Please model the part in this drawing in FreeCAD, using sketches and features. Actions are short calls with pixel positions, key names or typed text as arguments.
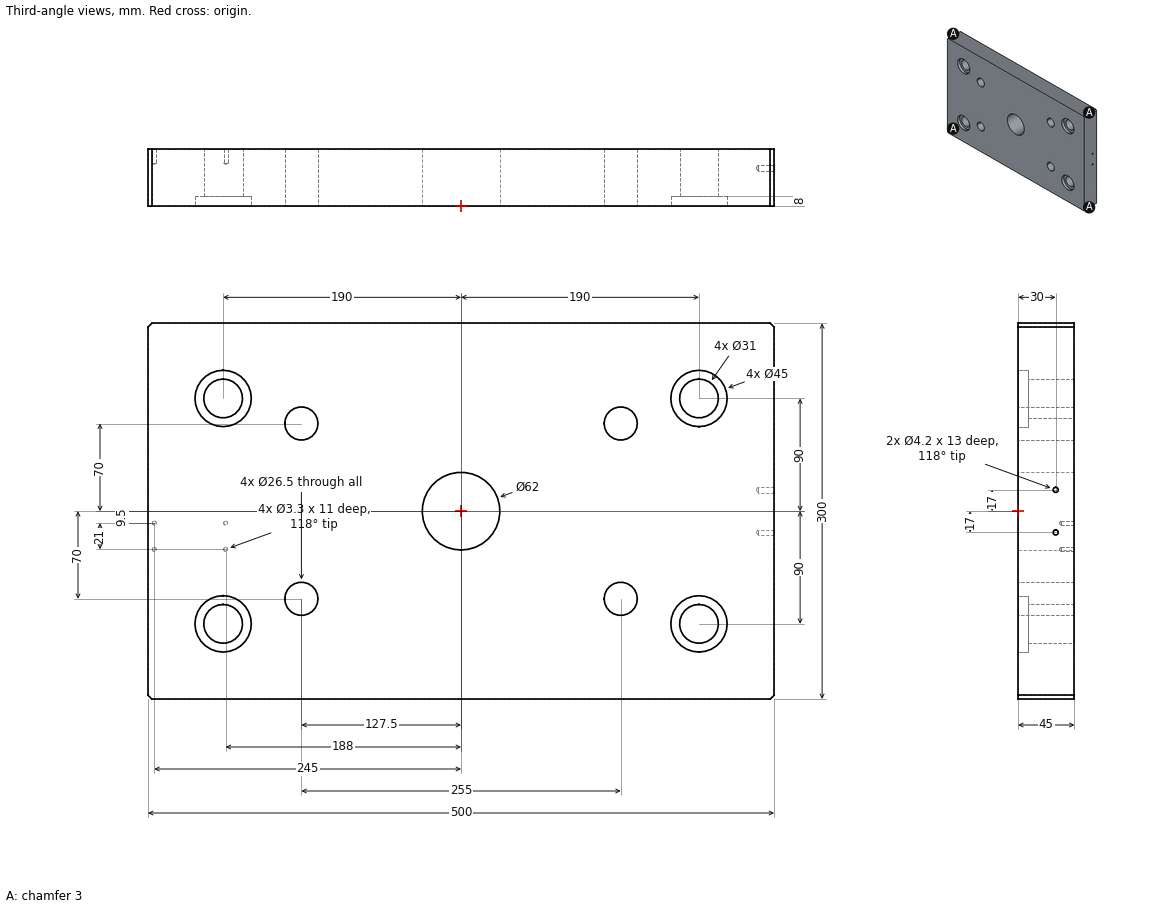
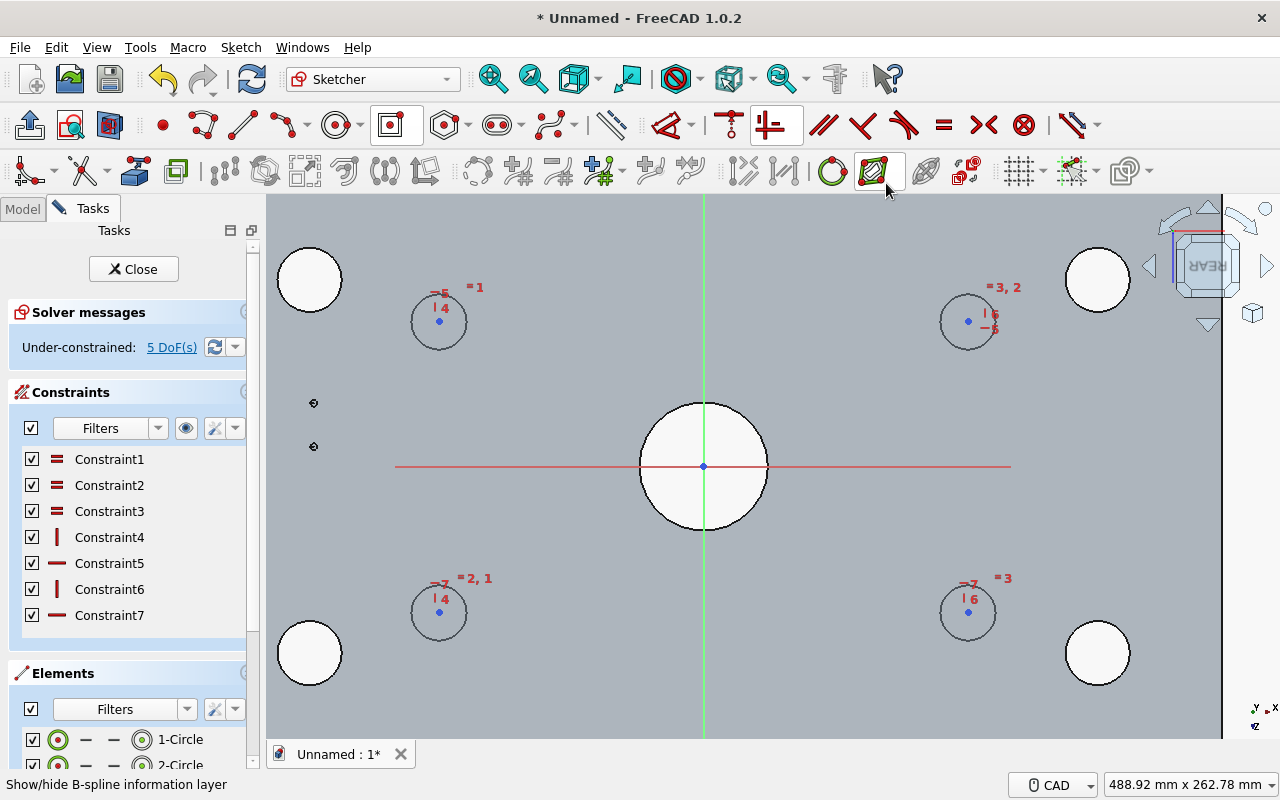
click(666, 126)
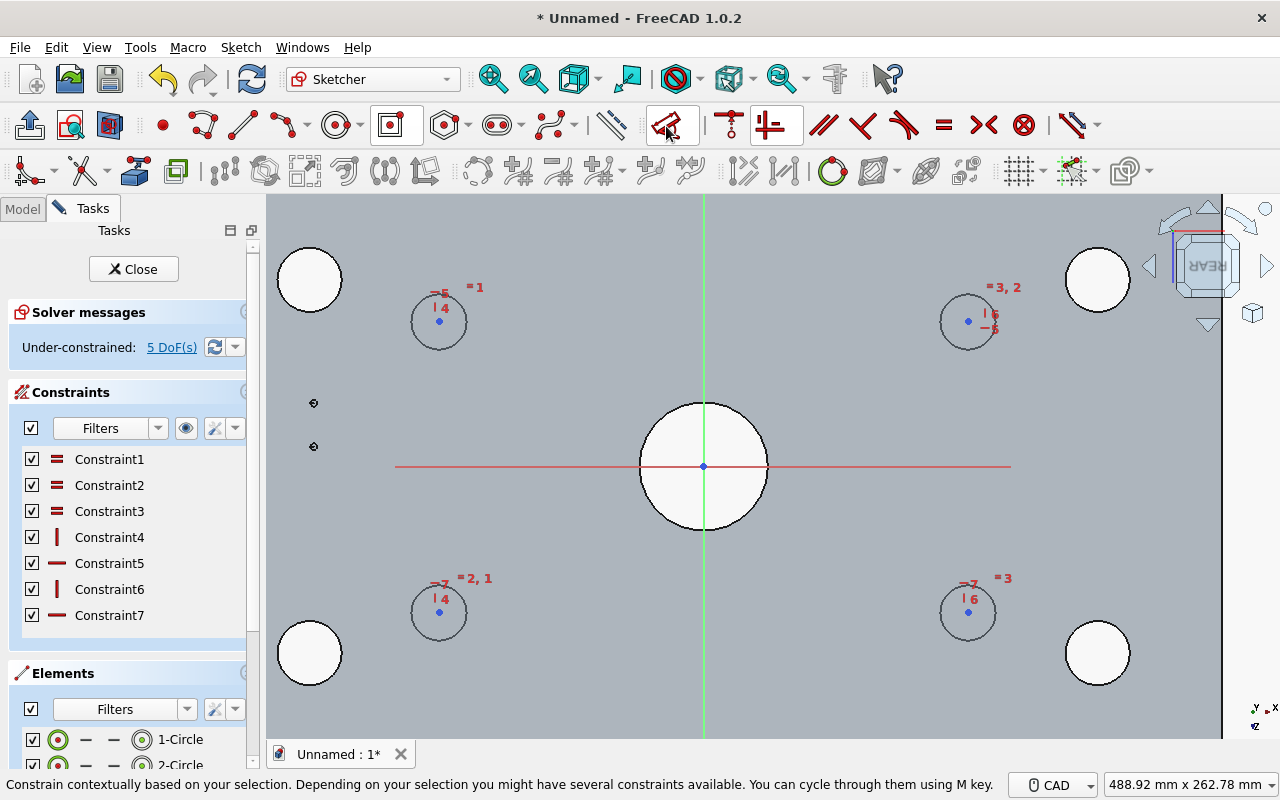
click(458, 302)
click(480, 279)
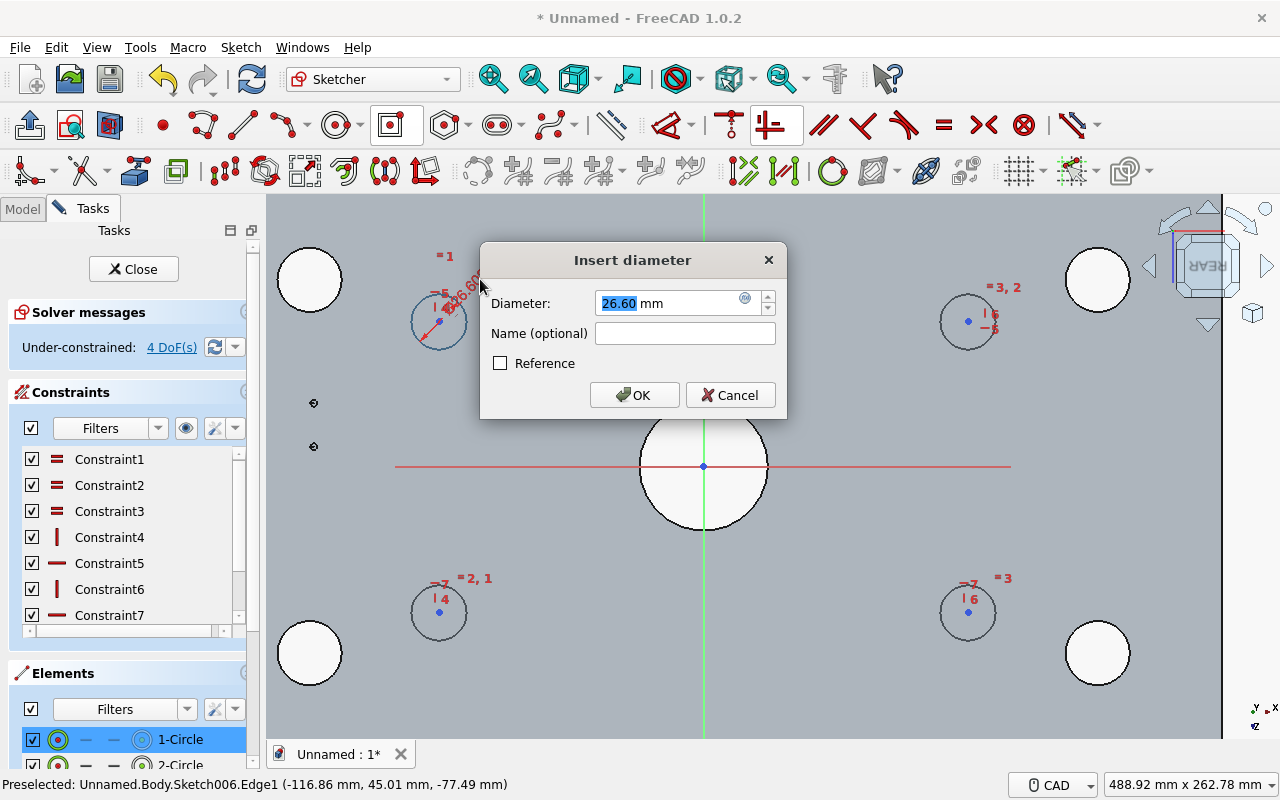
text(26.5)
key(Return)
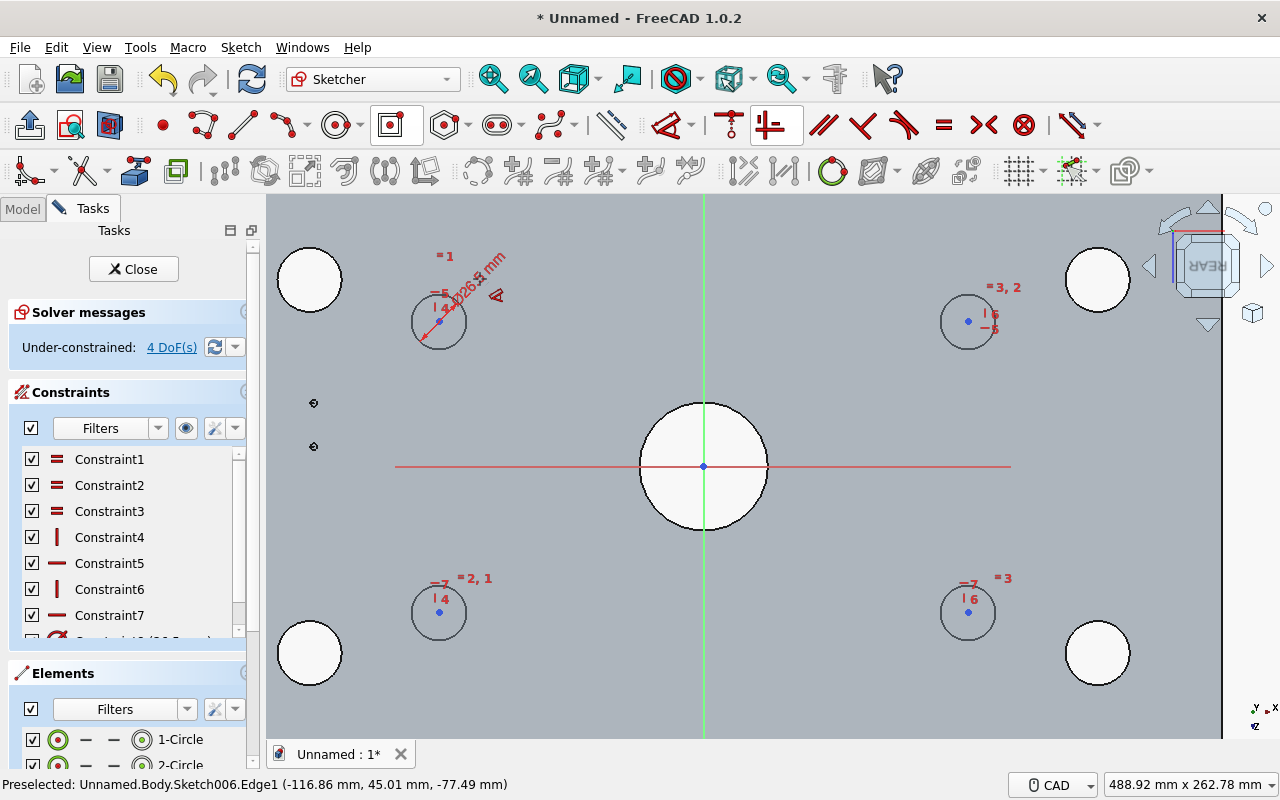
click(439, 322)
click(405, 394)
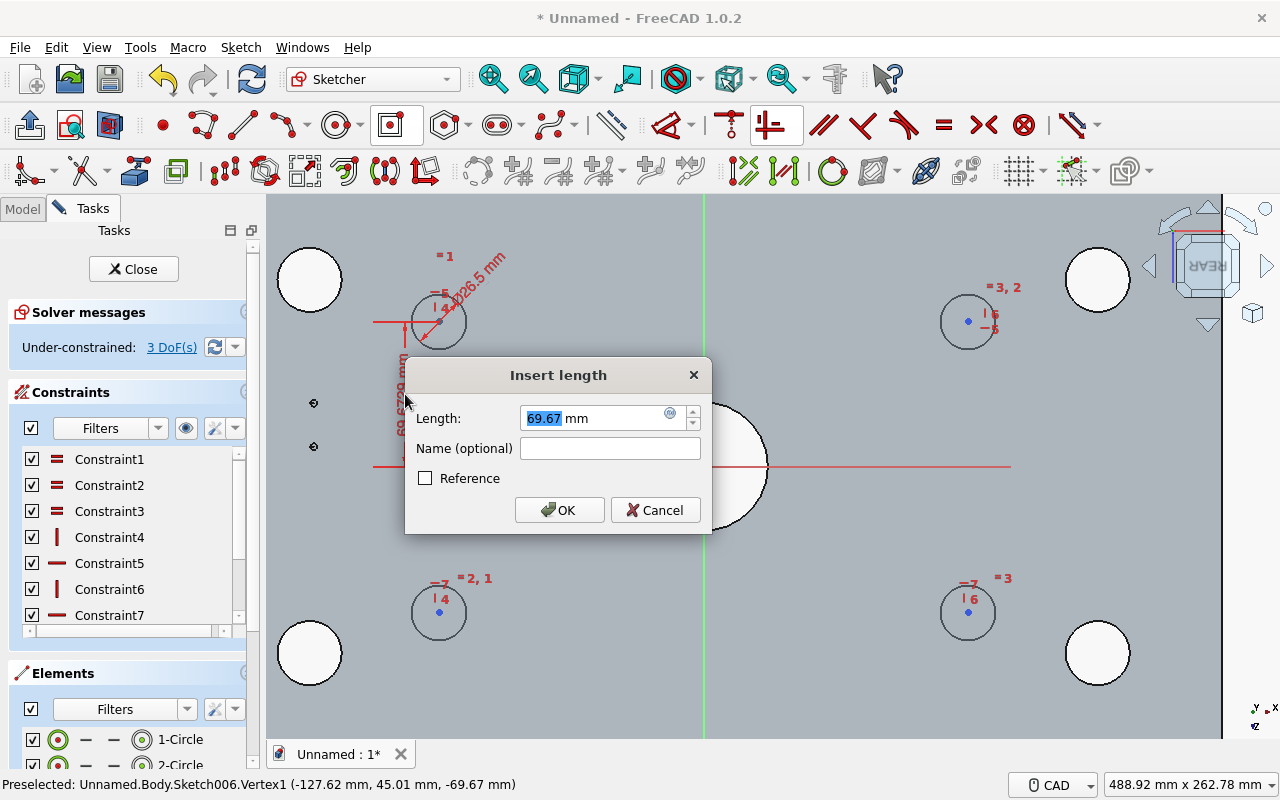
text(70)
key(Return)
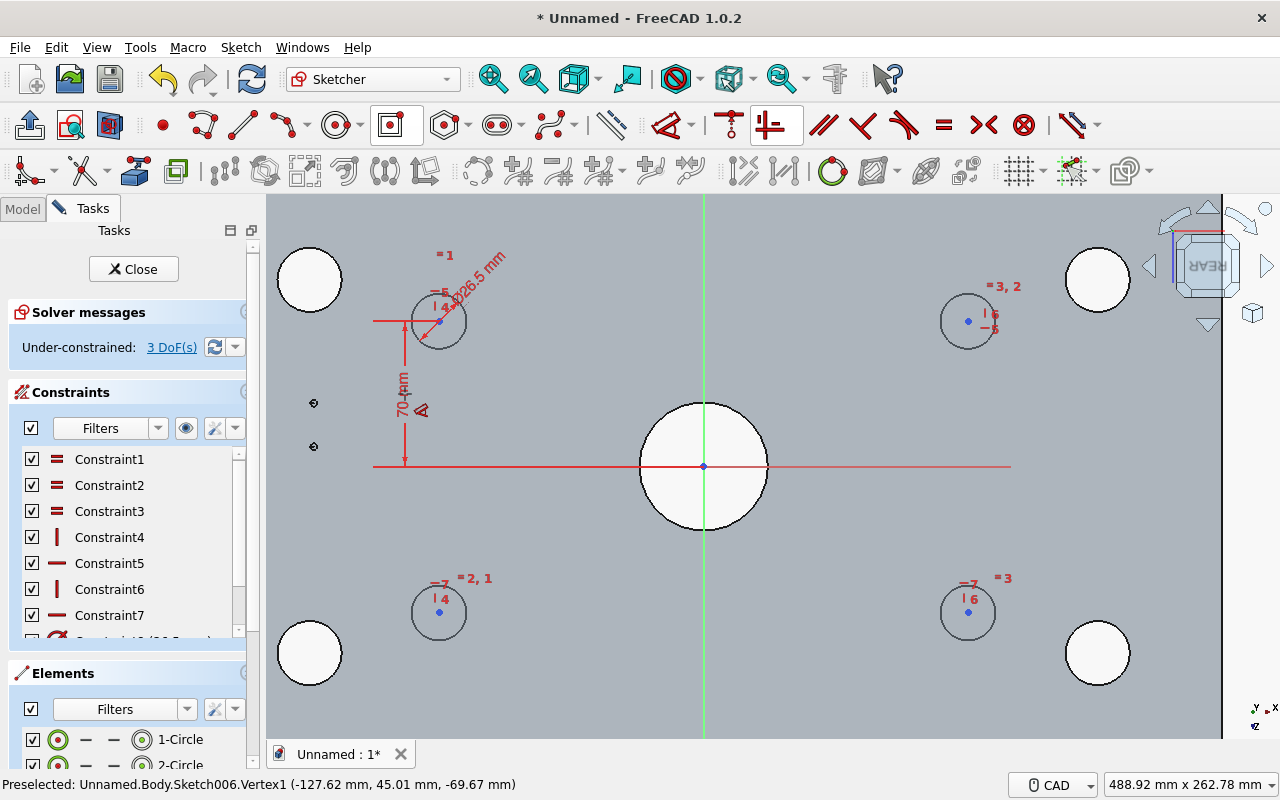
click(439, 613)
click(405, 540)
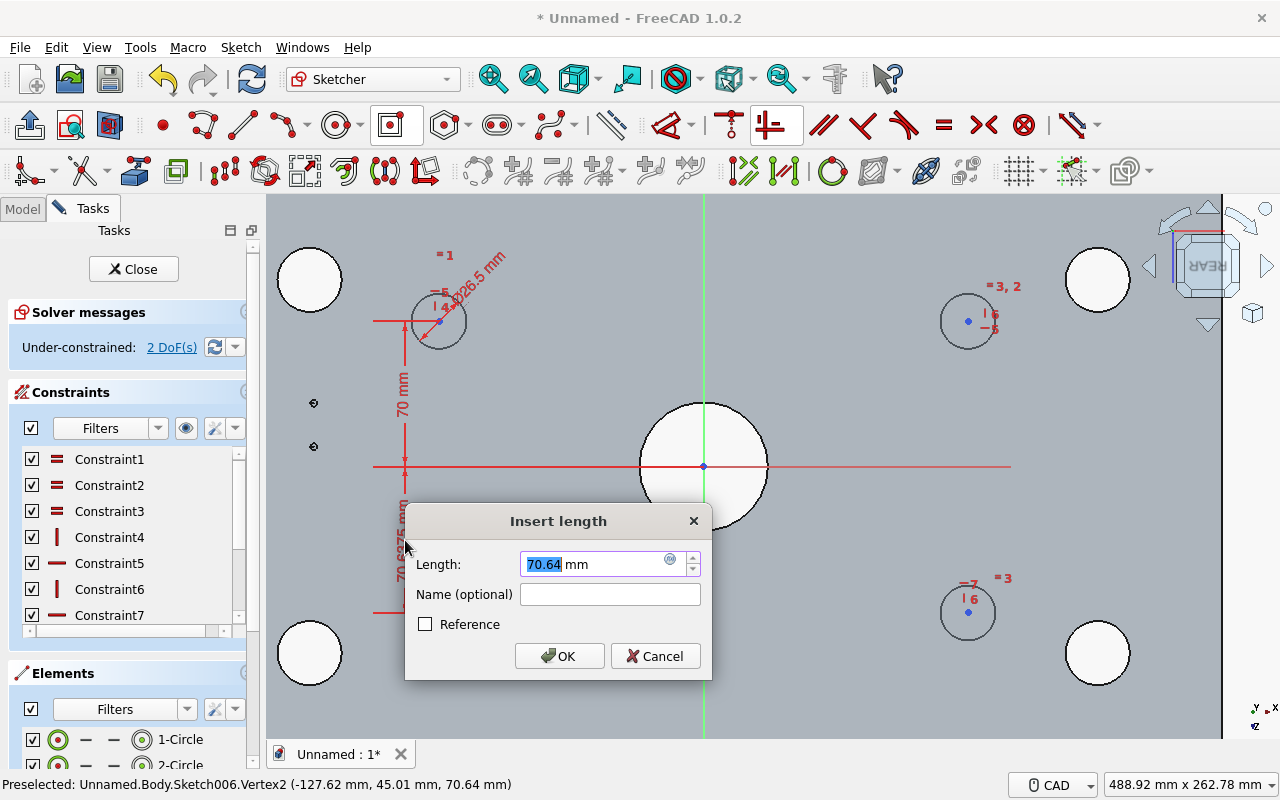
text(70)
key(Return)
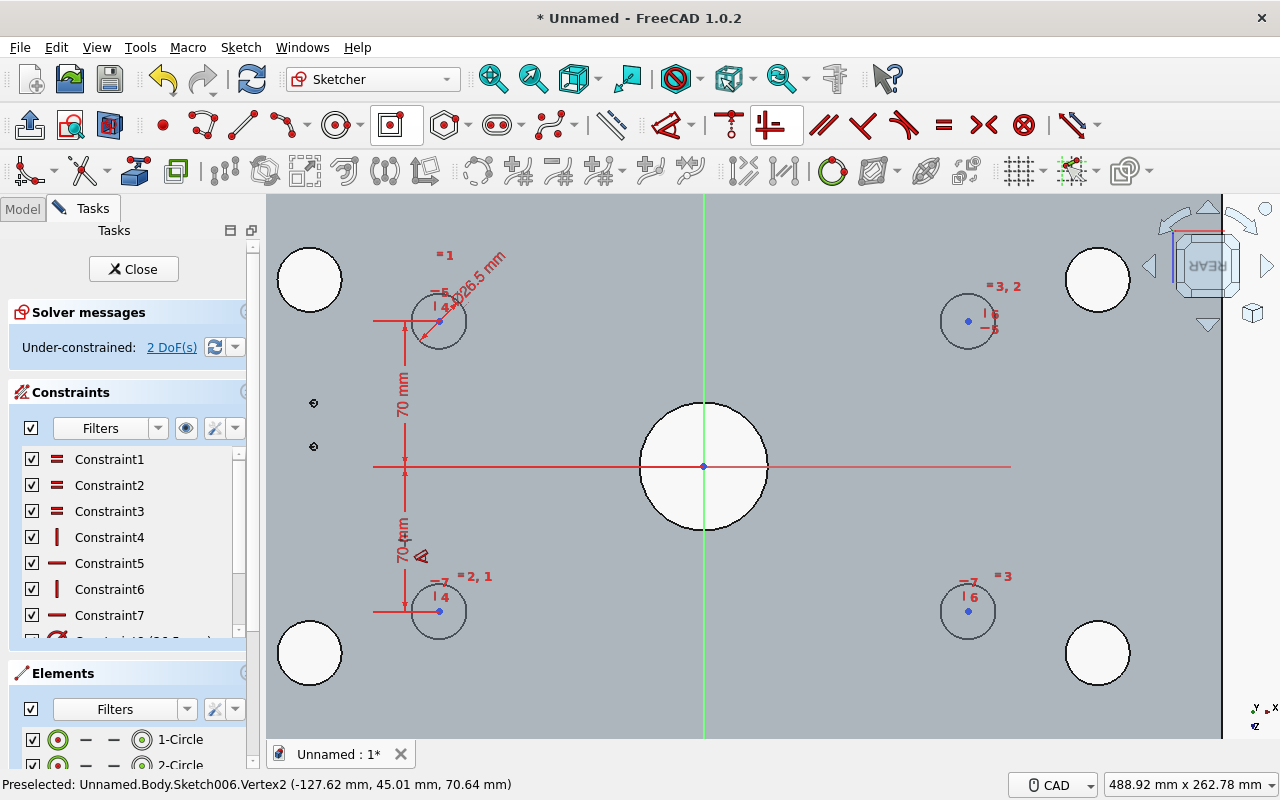
click(439, 321)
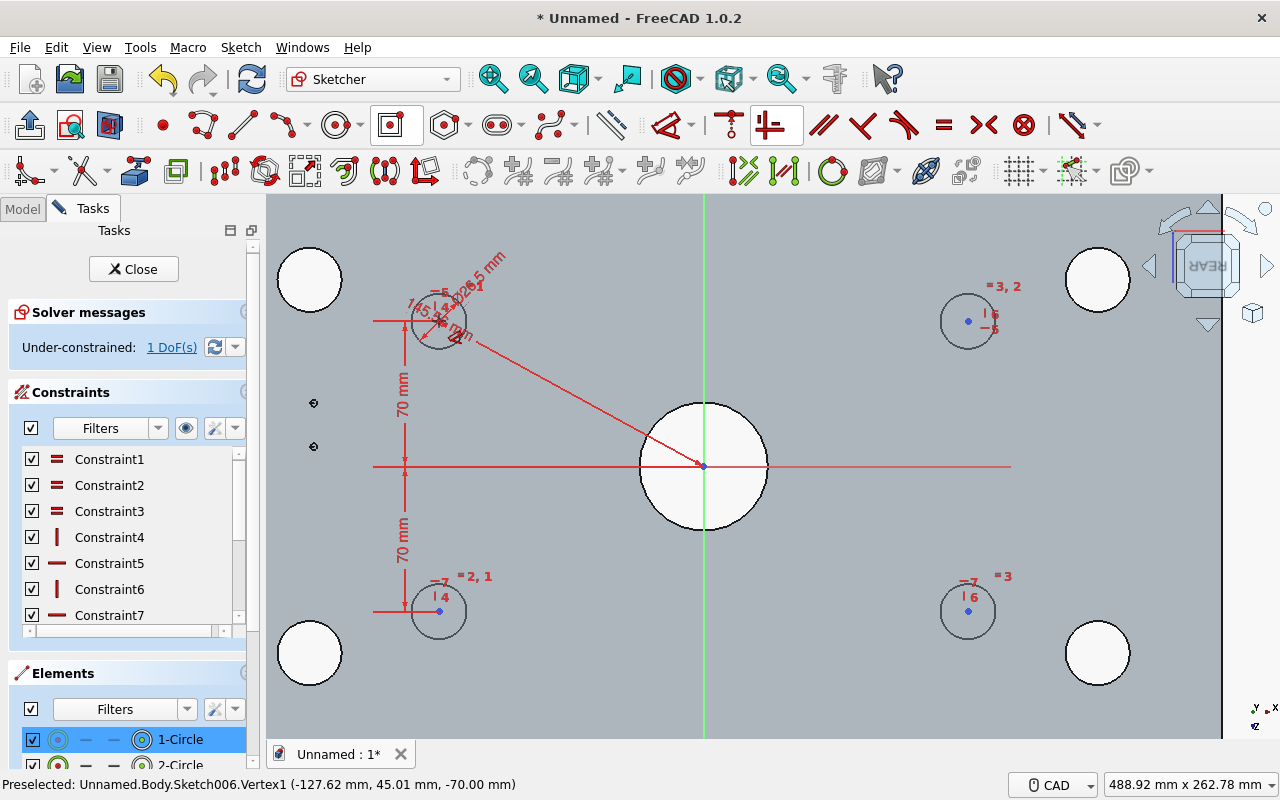
click(968, 321)
click(582, 287)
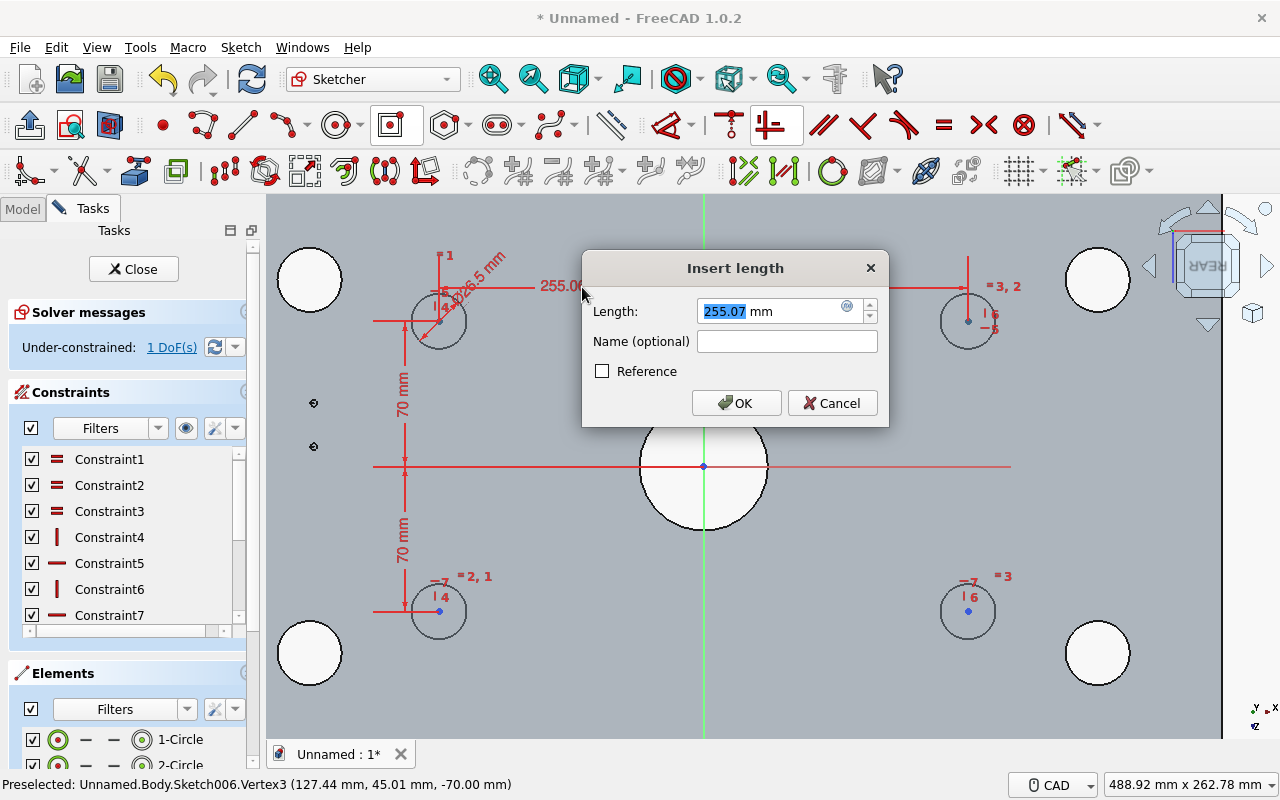
text(255)
key(Return)